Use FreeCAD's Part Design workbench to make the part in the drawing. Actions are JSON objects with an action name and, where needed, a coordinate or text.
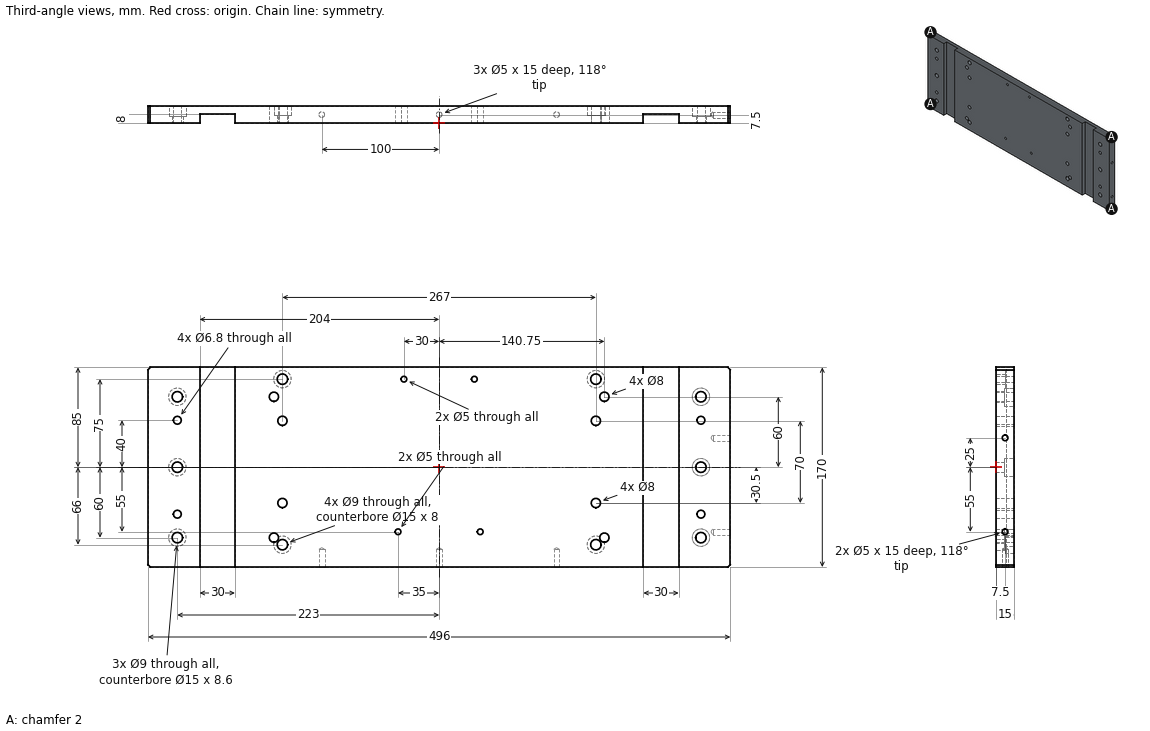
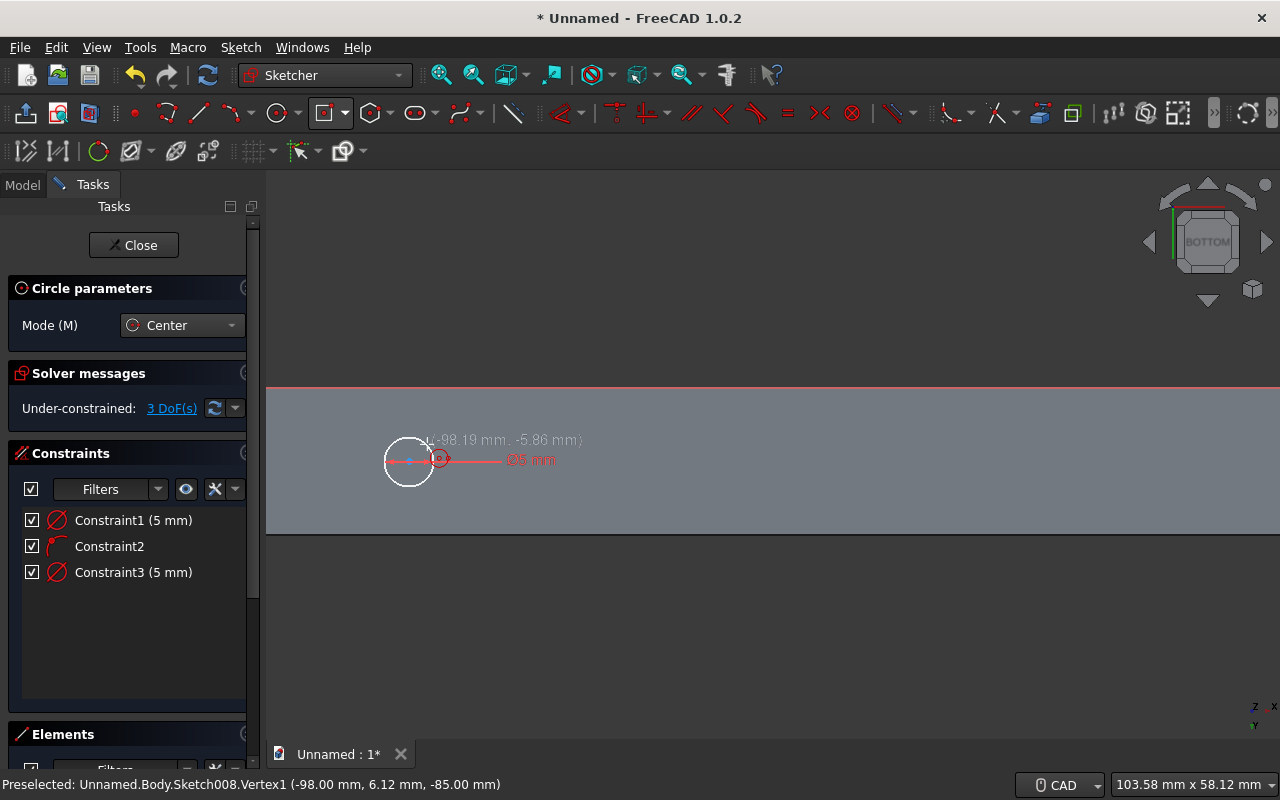
{"action": "scroll", "coordinate": [410, 462], "scroll_direction": "down", "scroll_amount": 6}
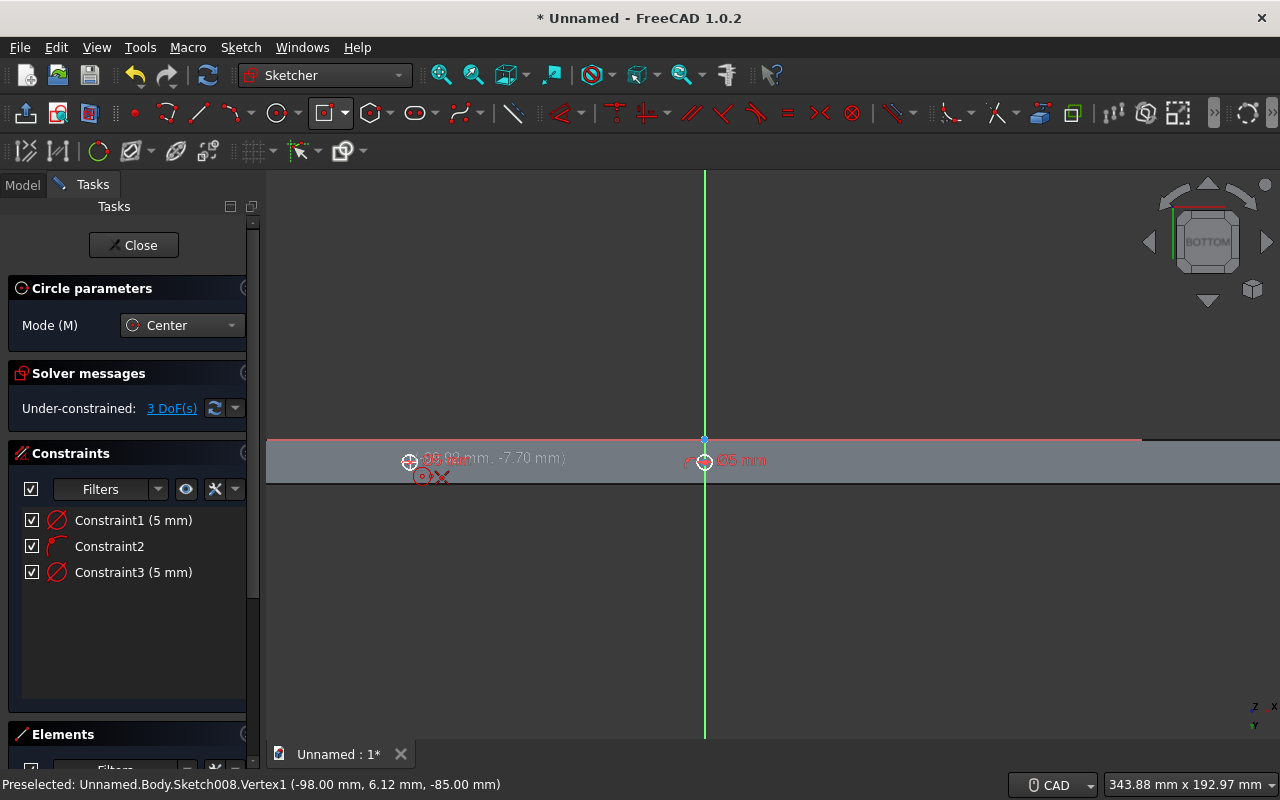
{"action": "scroll", "coordinate": [1000, 462], "scroll_direction": "up", "scroll_amount": 6}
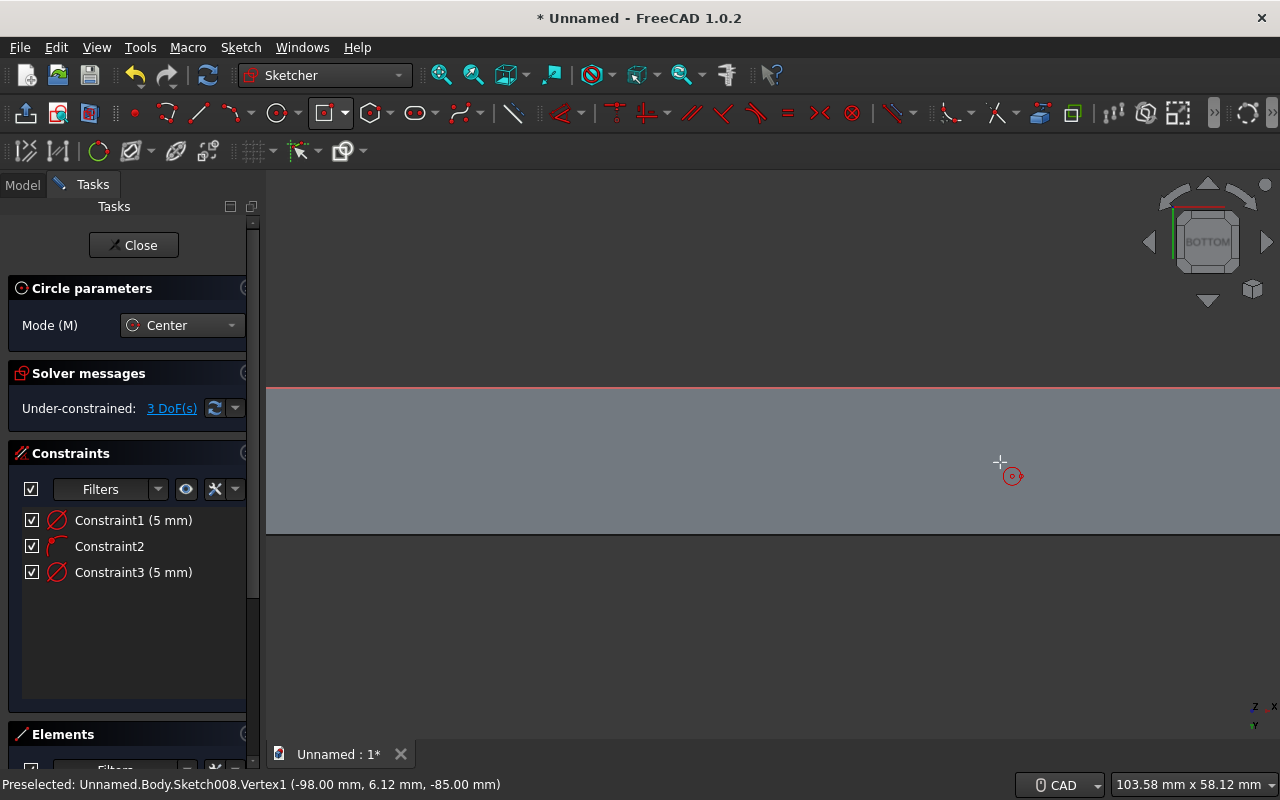
{"action": "left_click", "coordinate": [997, 461]}
{"action": "mouse_move", "coordinate": [1014, 444]}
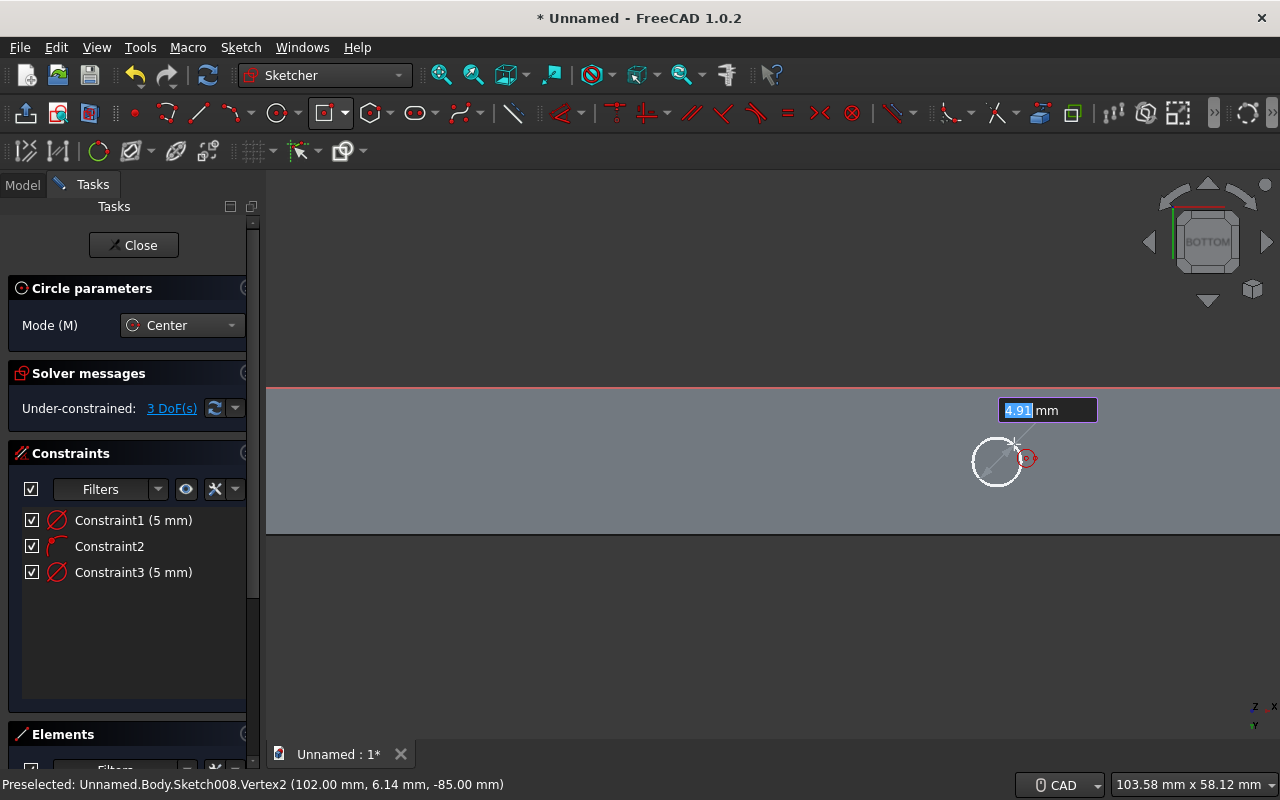
{"action": "type", "text": "5"}
{"action": "key", "text": "Return"}
{"action": "key", "text": "Escape"}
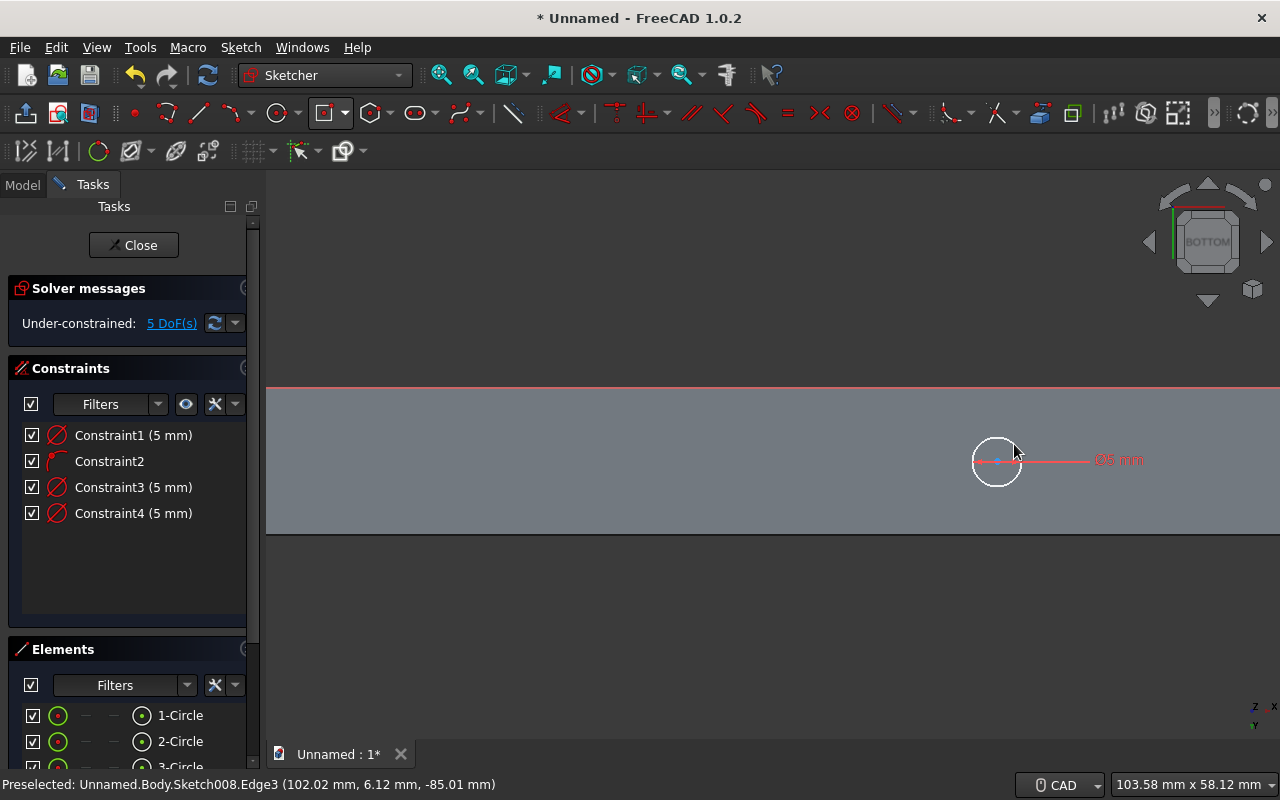
{"action": "scroll", "coordinate": [1000, 462], "scroll_direction": "down", "scroll_amount": 6}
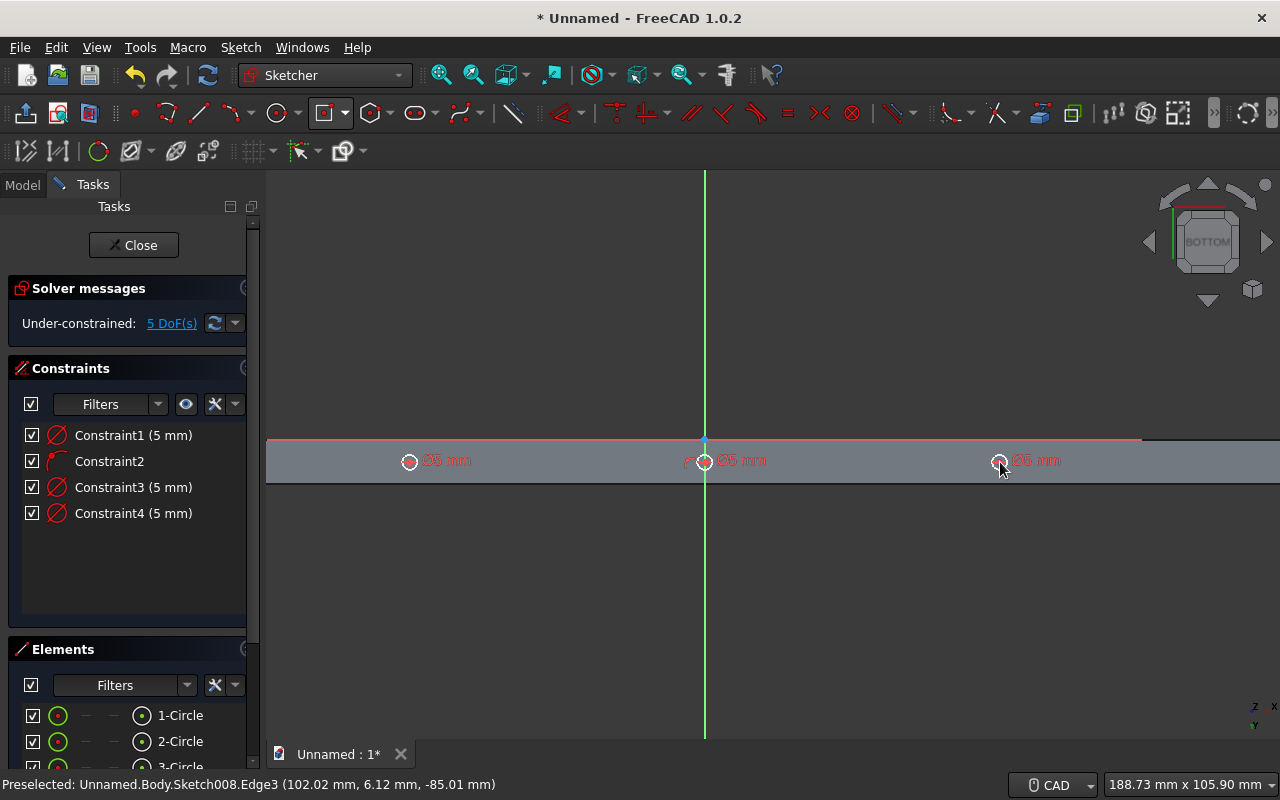
{"action": "left_click", "coordinate": [410, 462]}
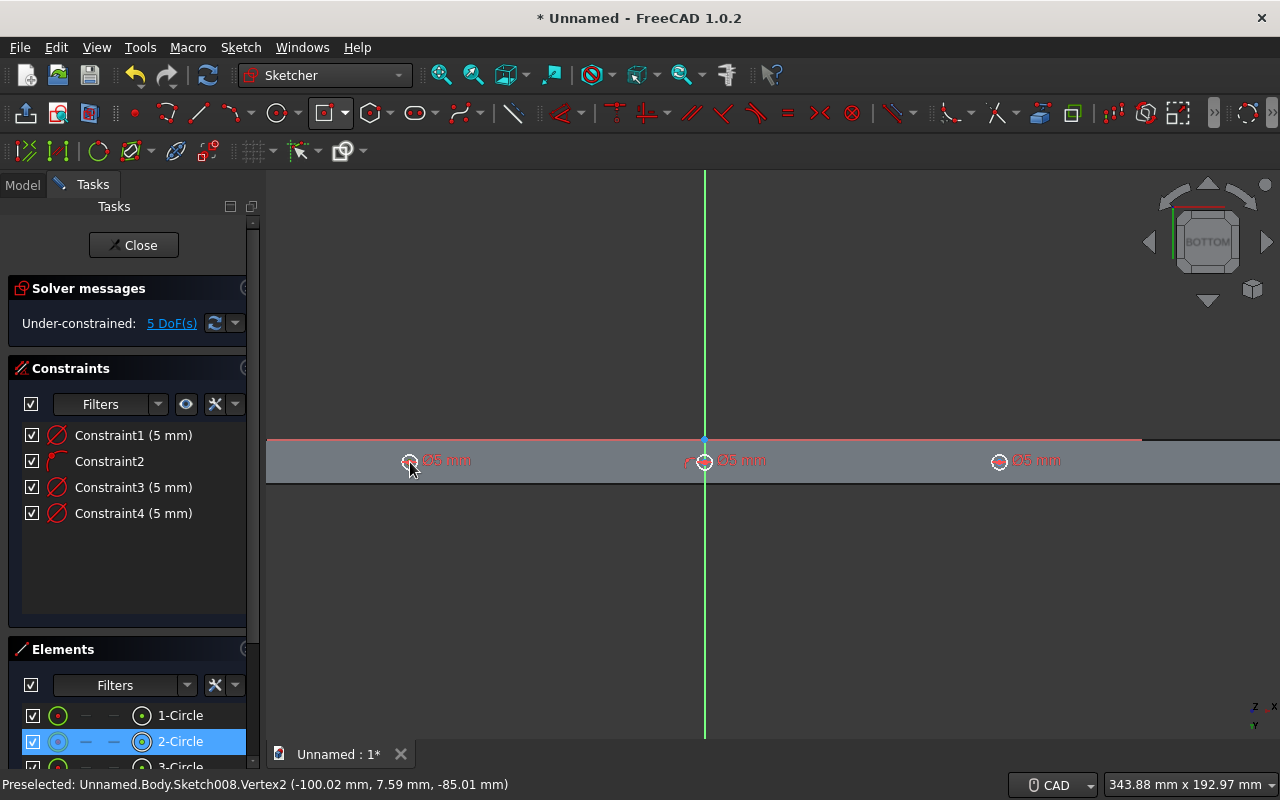
{"action": "left_click", "coordinate": [1000, 462]}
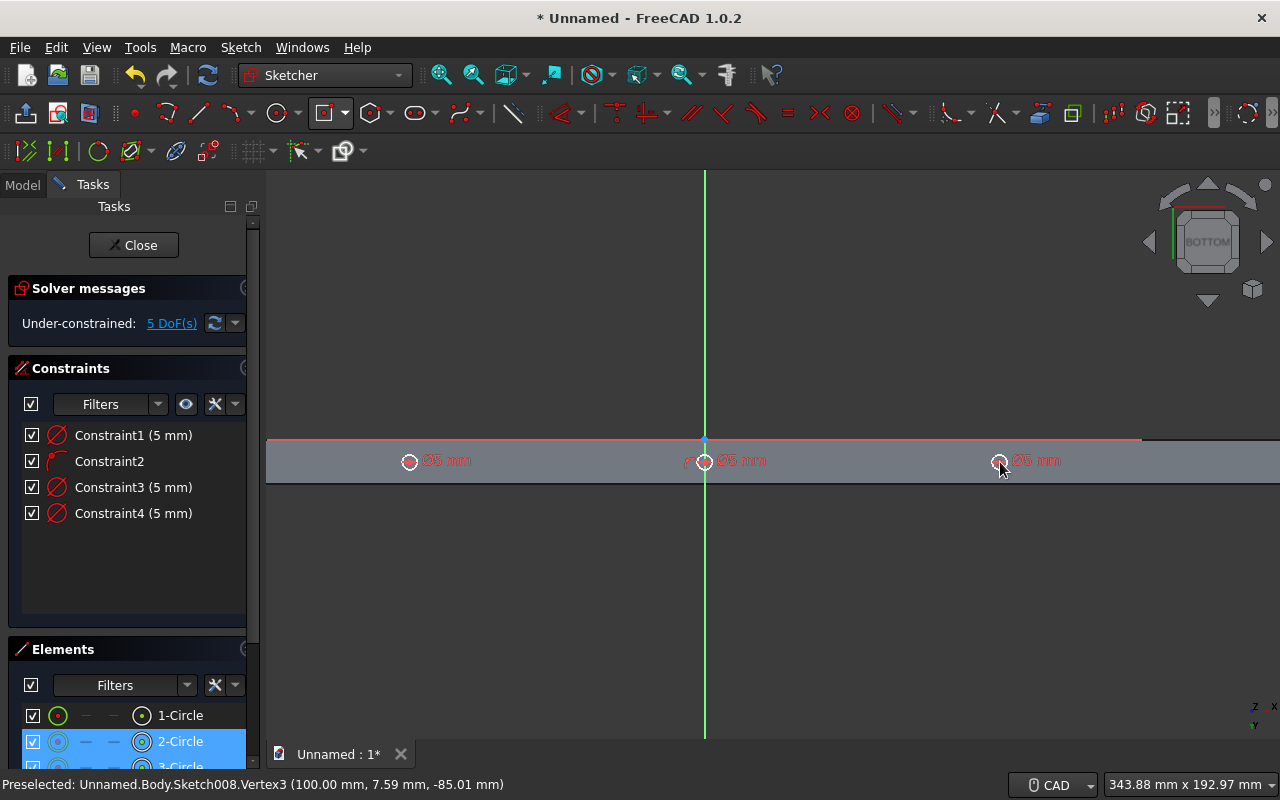
{"action": "left_click", "coordinate": [705, 674]}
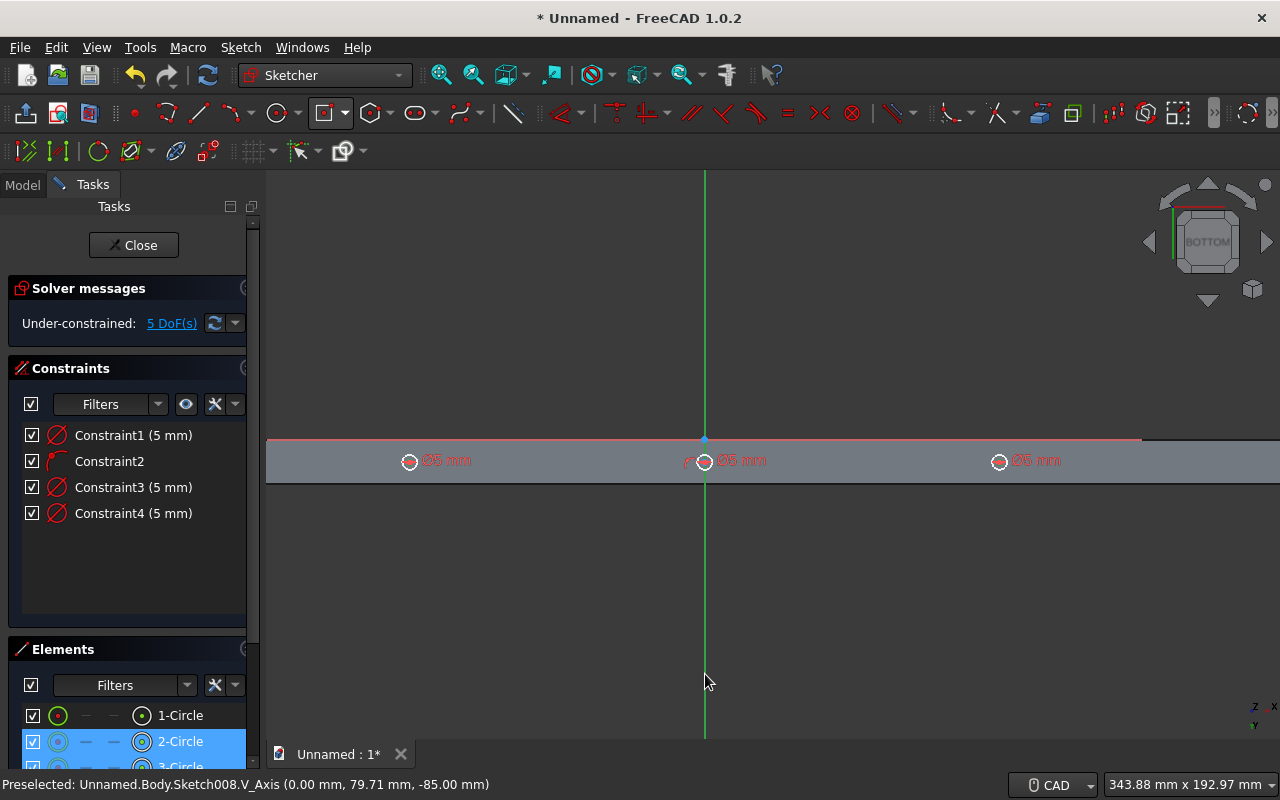
{"action": "left_click", "coordinate": [820, 114]}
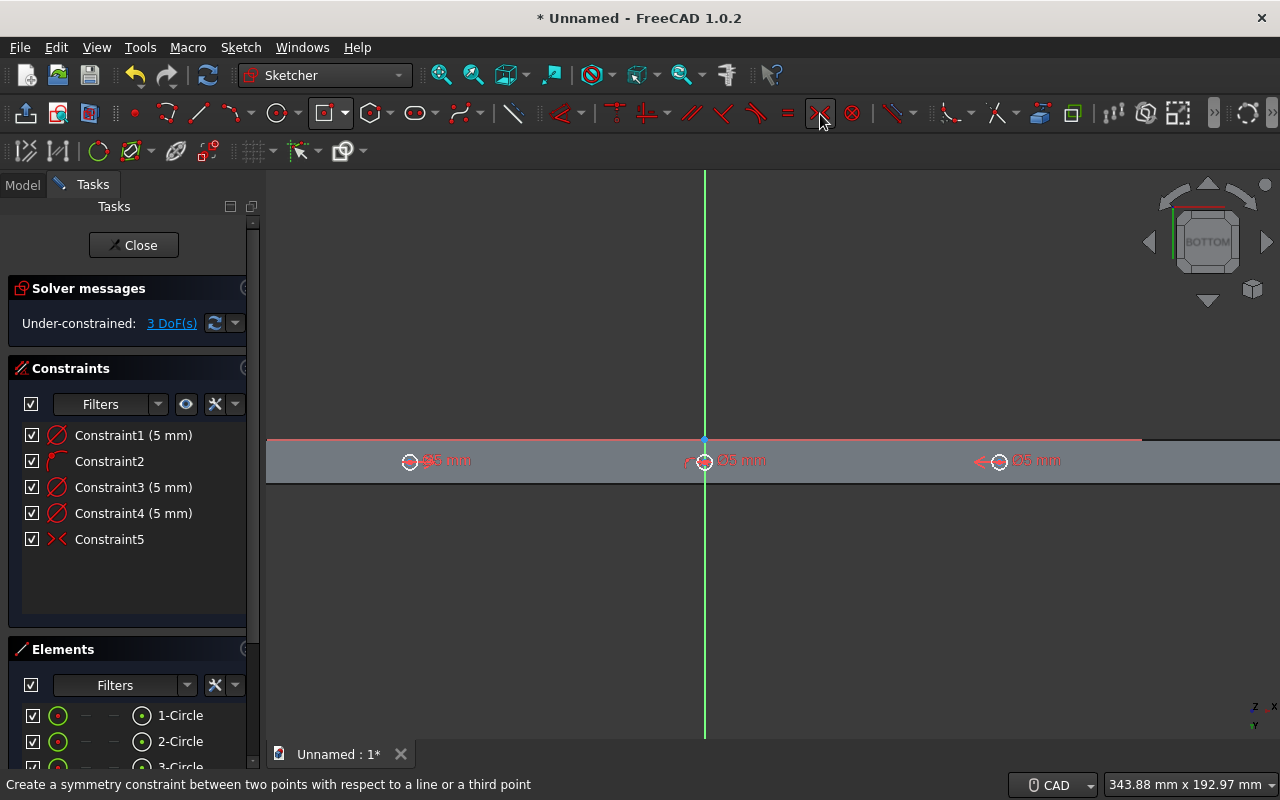
{"action": "left_click", "coordinate": [560, 114]}